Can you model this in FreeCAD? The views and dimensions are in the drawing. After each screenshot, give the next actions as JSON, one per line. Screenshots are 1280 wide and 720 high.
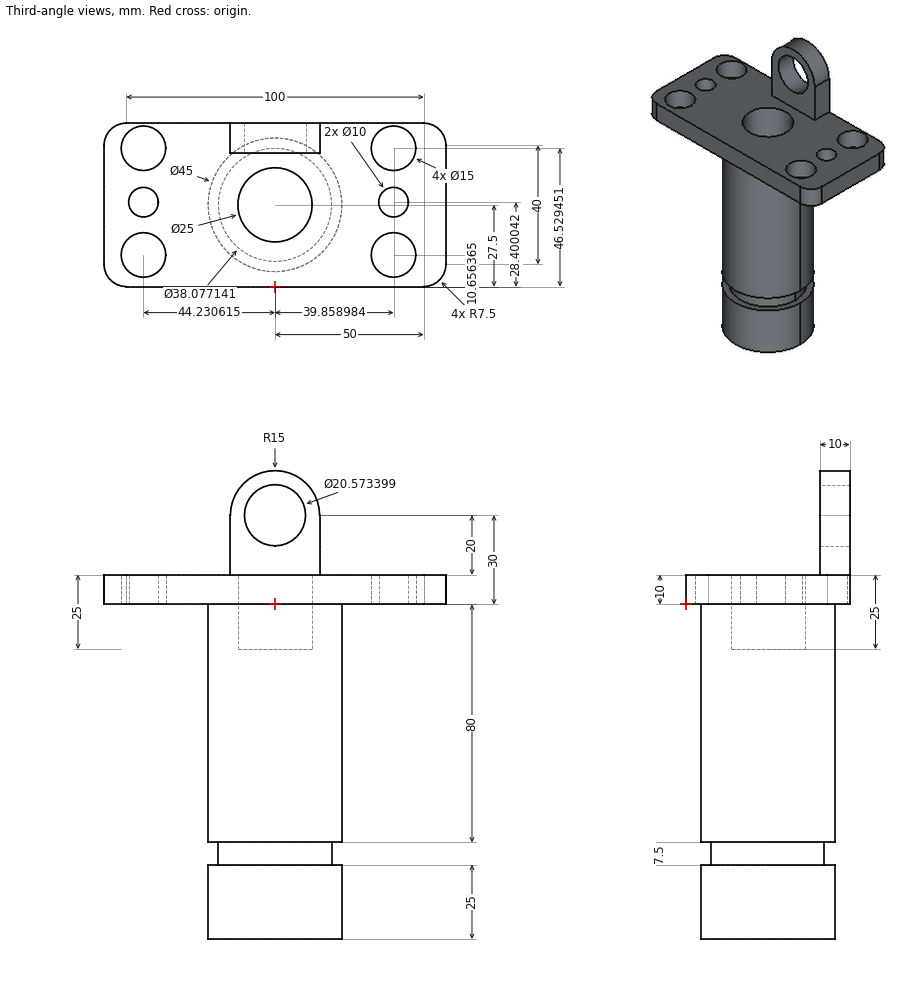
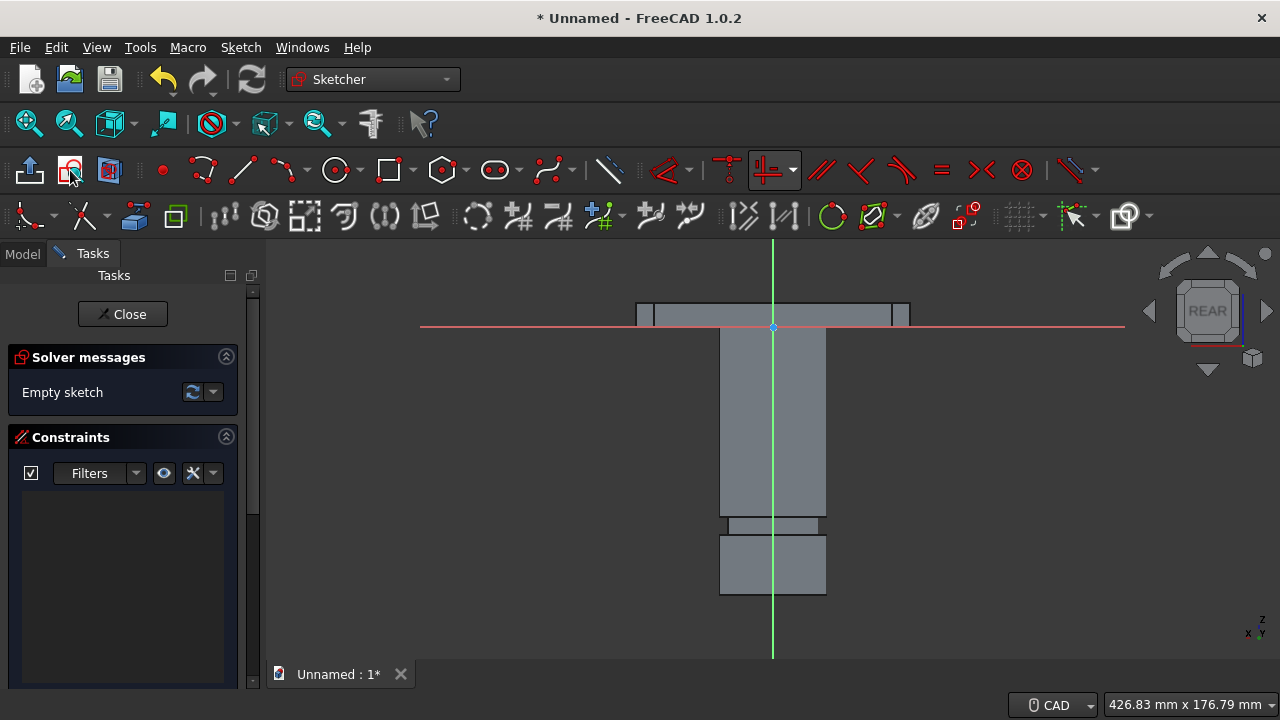
{"action": "scroll", "coordinate": [704, 449], "scroll_direction": "down", "scroll_amount": 5}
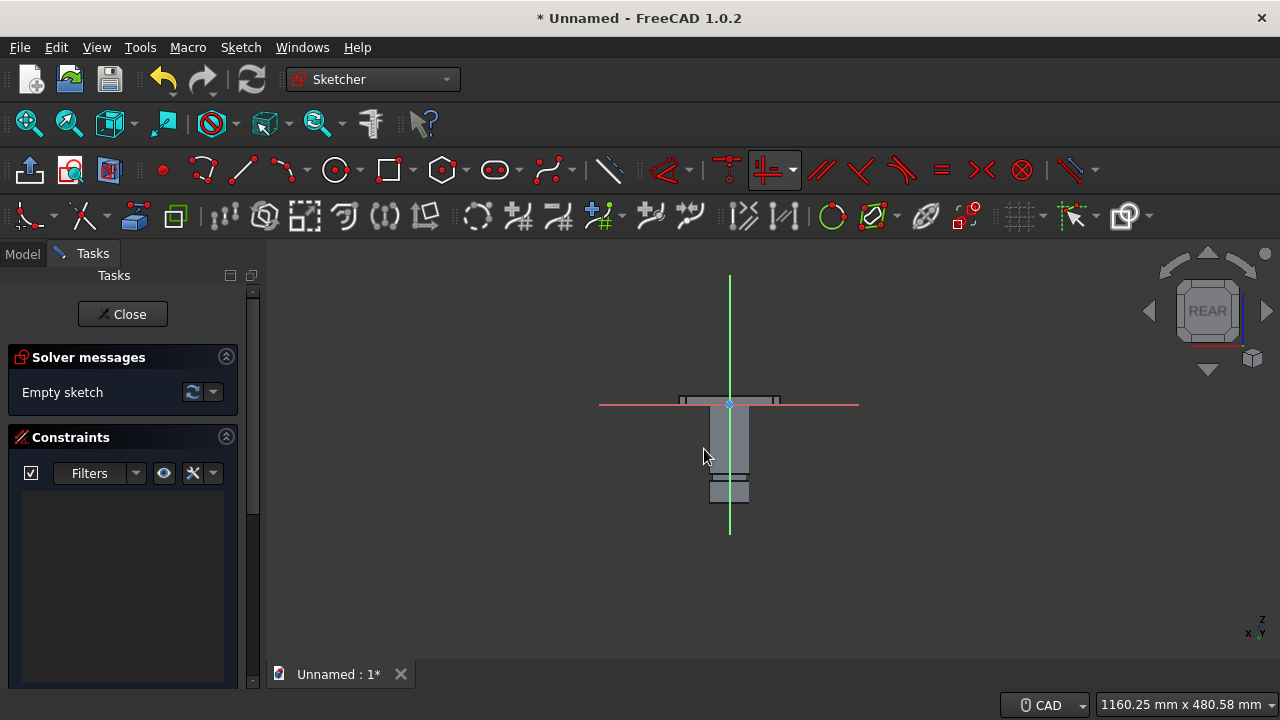
{"action": "scroll", "coordinate": [735, 372], "scroll_direction": "up", "scroll_amount": 9}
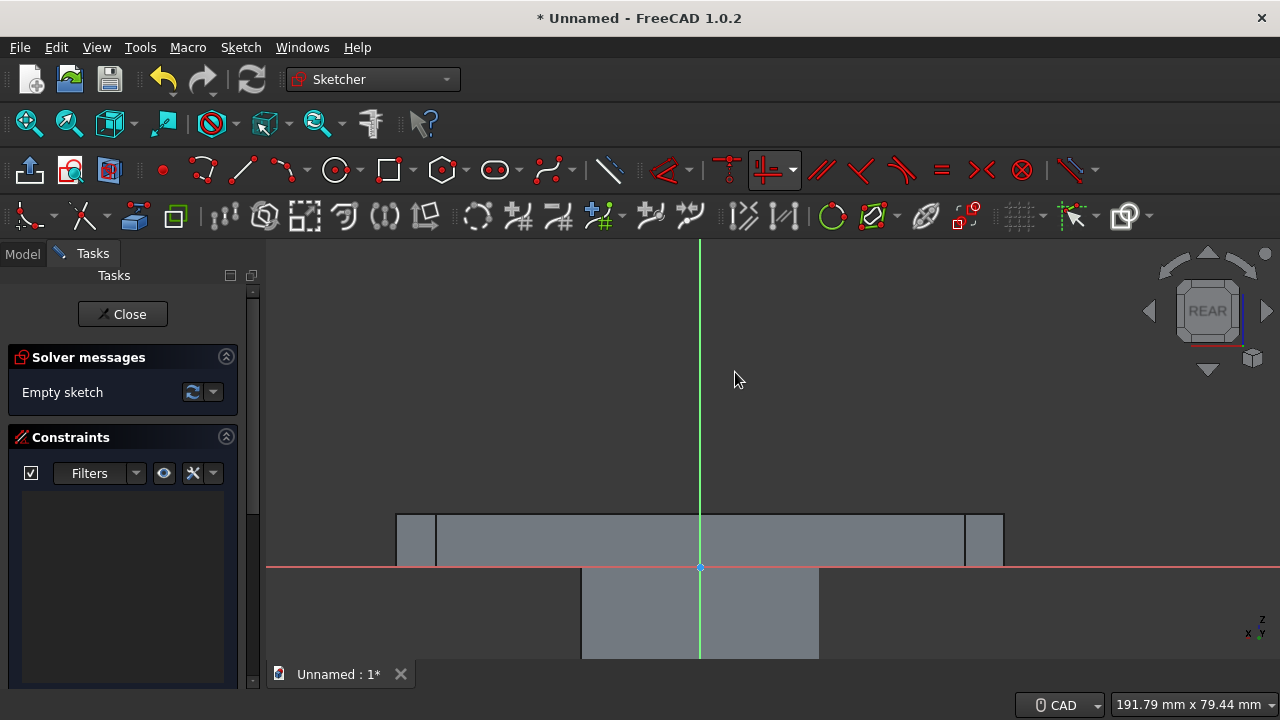
{"action": "left_click", "coordinate": [204, 170]}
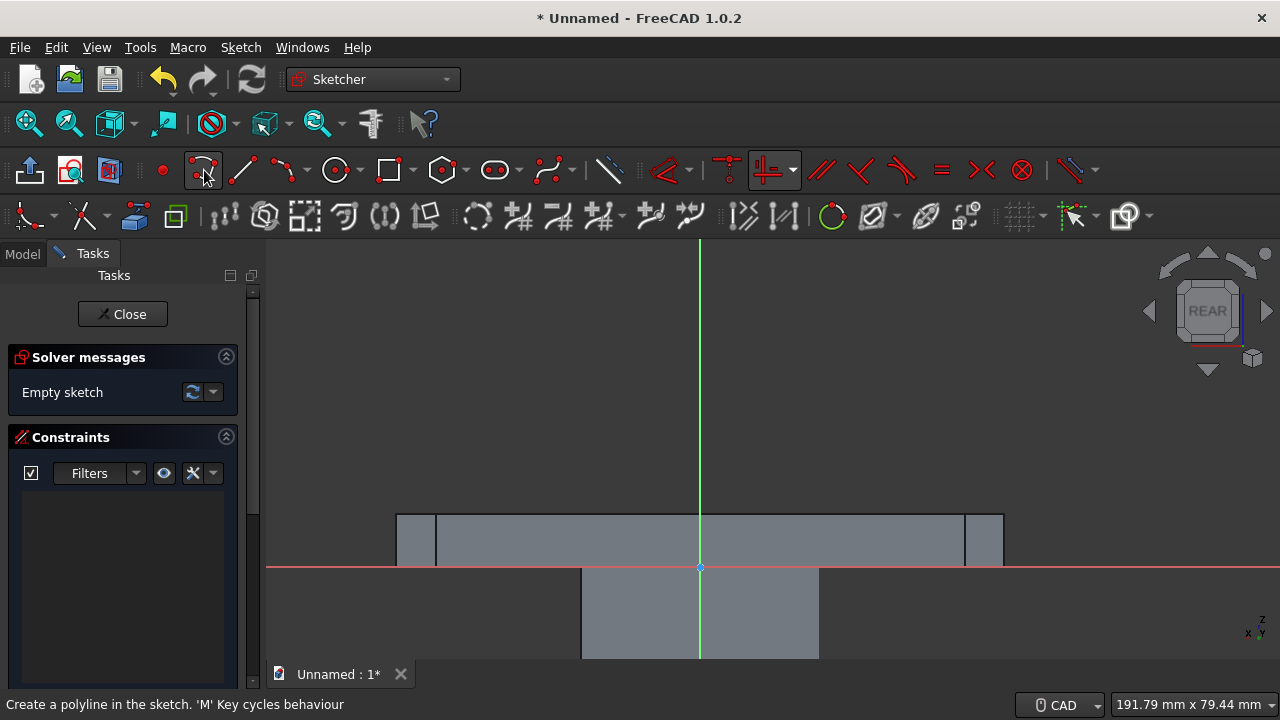
{"action": "left_click", "coordinate": [621, 409]}
{"action": "left_click", "coordinate": [621, 514]}
{"action": "left_click", "coordinate": [780, 514]}
{"action": "left_click", "coordinate": [780, 409]}
{"action": "right_click", "coordinate": [780, 409]}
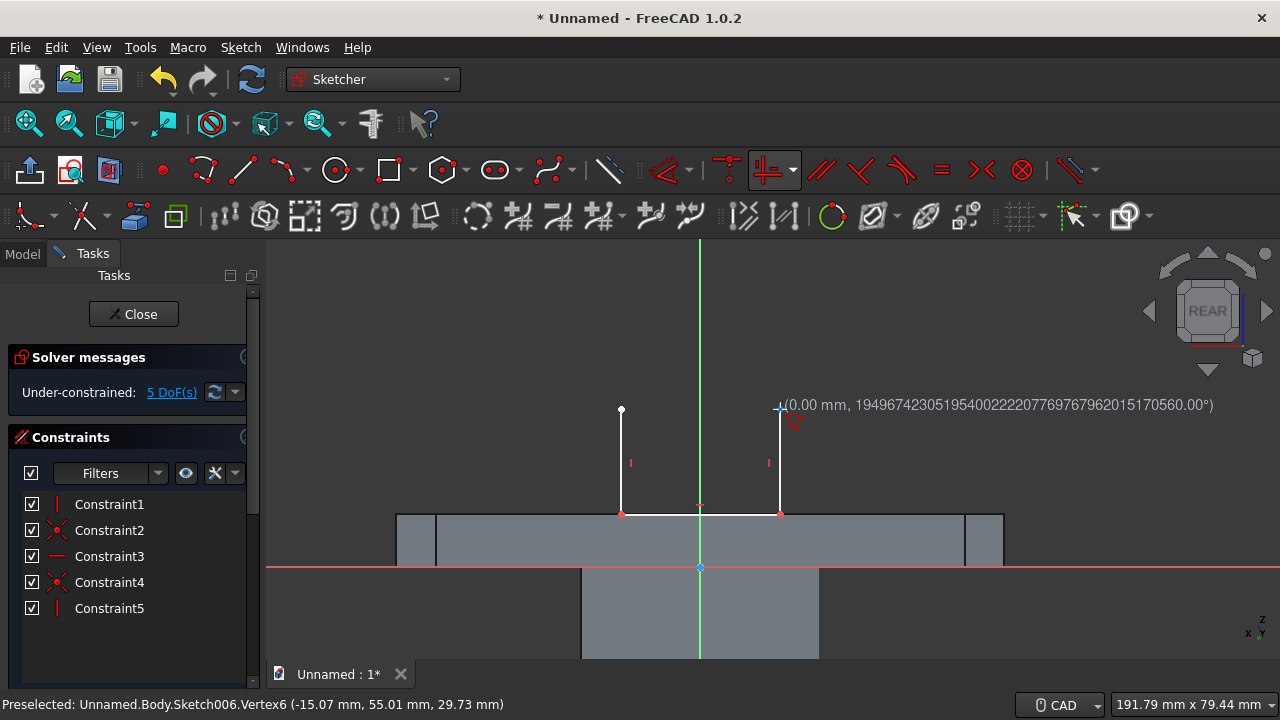
{"action": "left_click", "coordinate": [284, 170]}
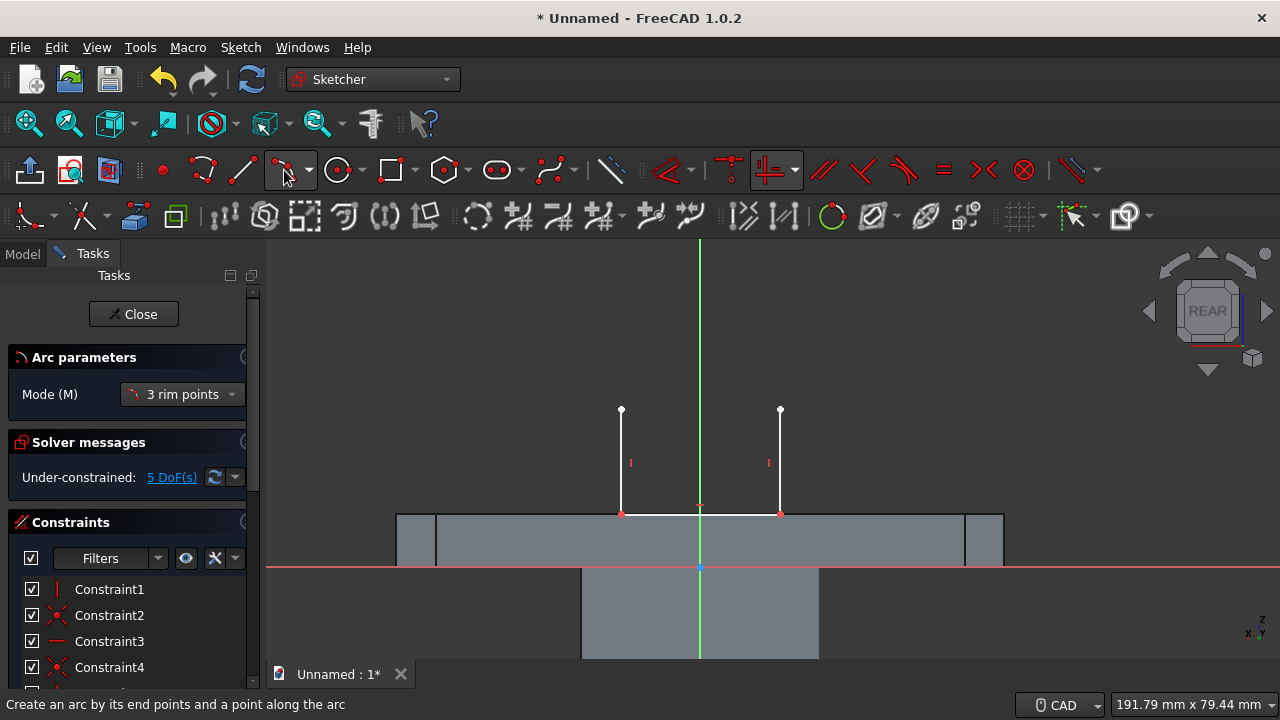
{"action": "left_click", "coordinate": [780, 410]}
{"action": "left_click", "coordinate": [621, 410]}
{"action": "left_click", "coordinate": [725, 333]}
{"action": "key", "text": "Escape"}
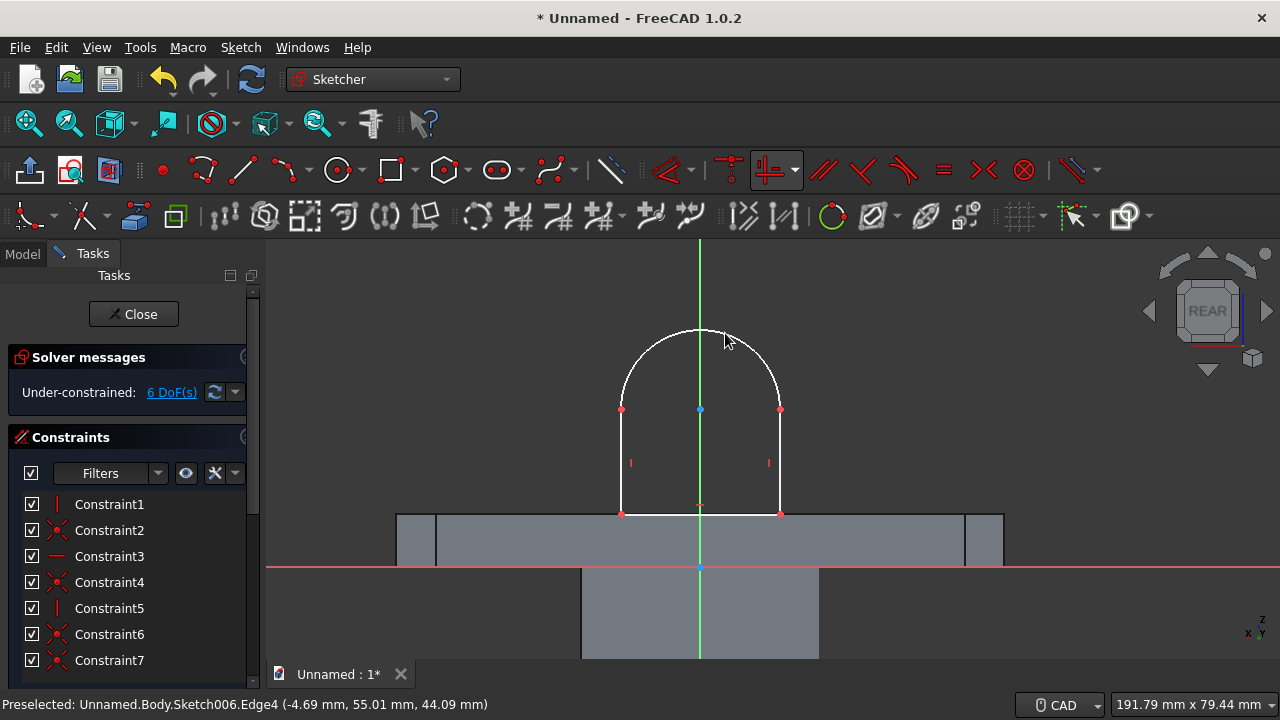
{"action": "left_click", "coordinate": [621, 442]}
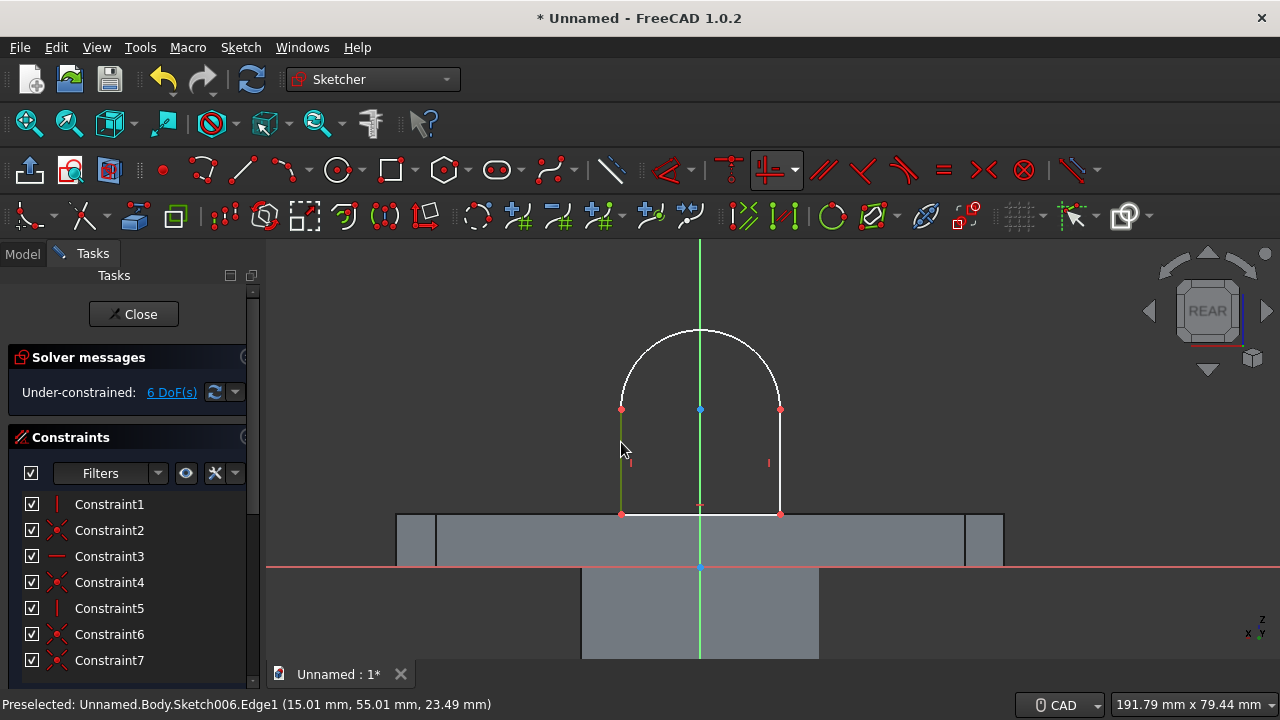
{"action": "left_click", "coordinate": [747, 345]}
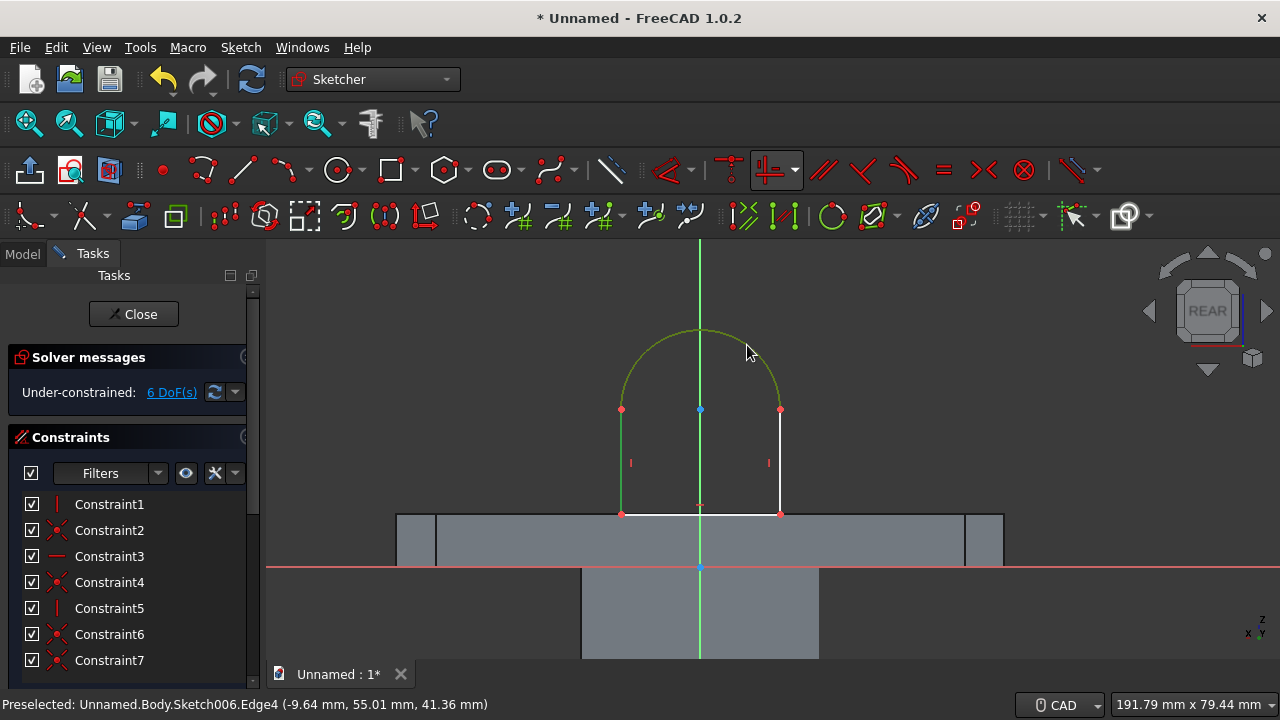
{"action": "key", "text": "t"}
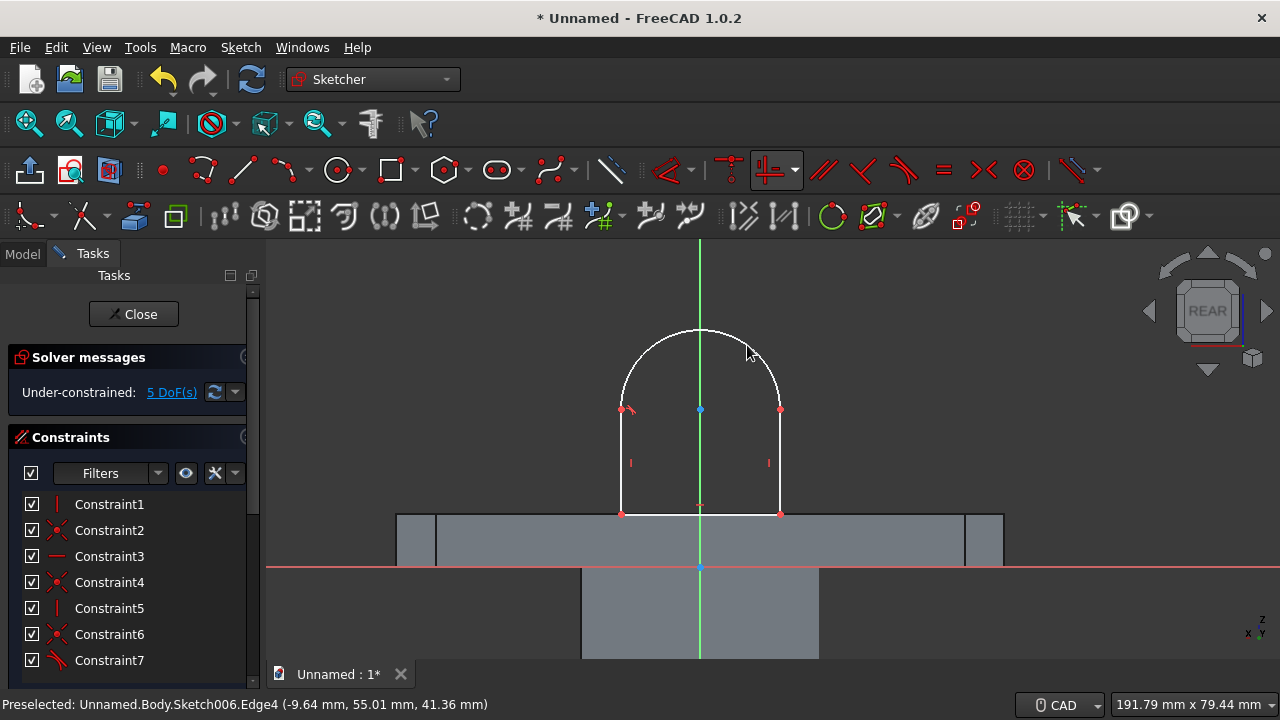
{"action": "left_click", "coordinate": [780, 483]}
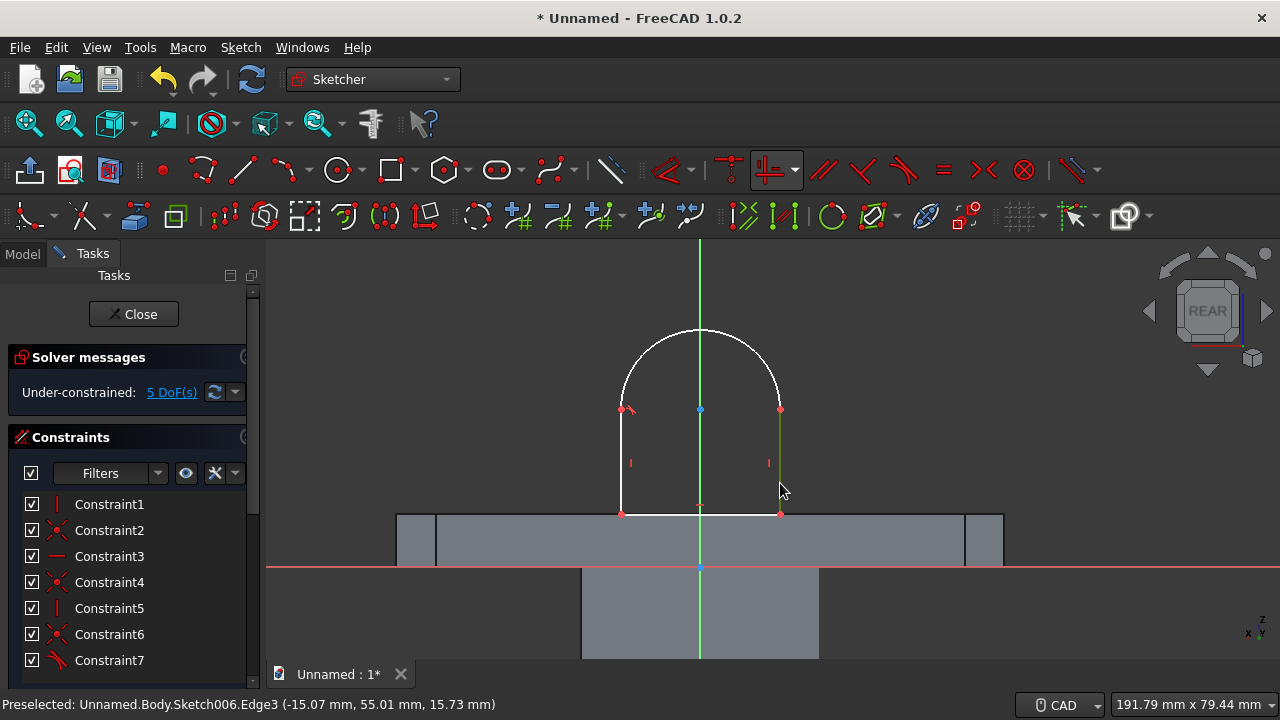
{"action": "left_click", "coordinate": [747, 345]}